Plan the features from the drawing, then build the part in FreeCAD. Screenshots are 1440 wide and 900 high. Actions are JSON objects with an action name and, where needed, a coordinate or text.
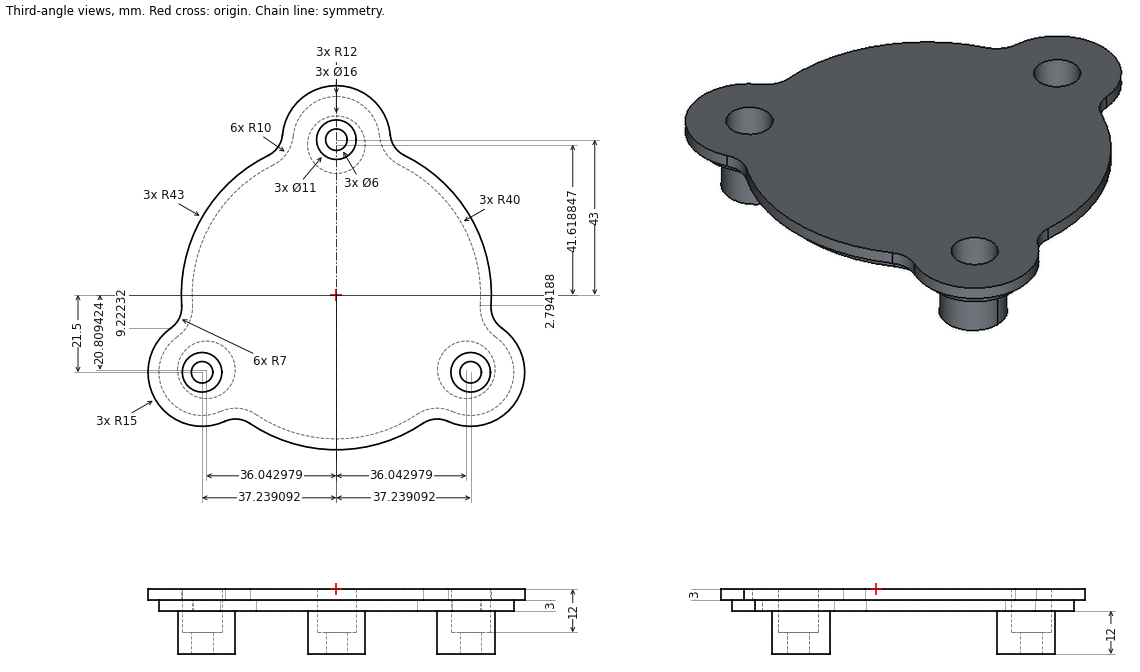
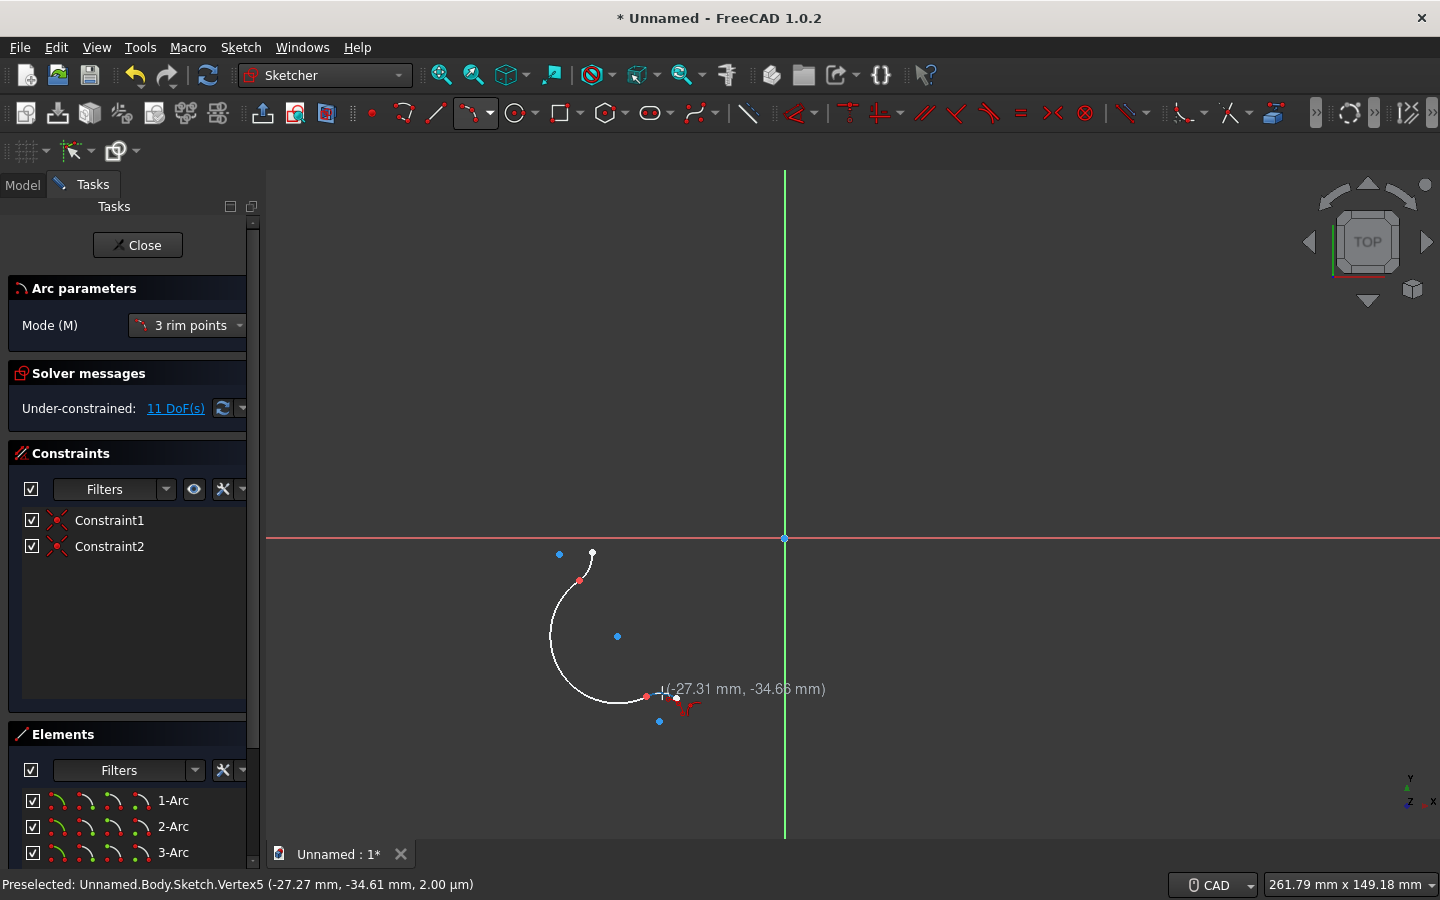
{"action": "left_click", "coordinate": [677, 699]}
{"action": "left_click", "coordinate": [893, 698]}
{"action": "left_click", "coordinate": [762, 730]}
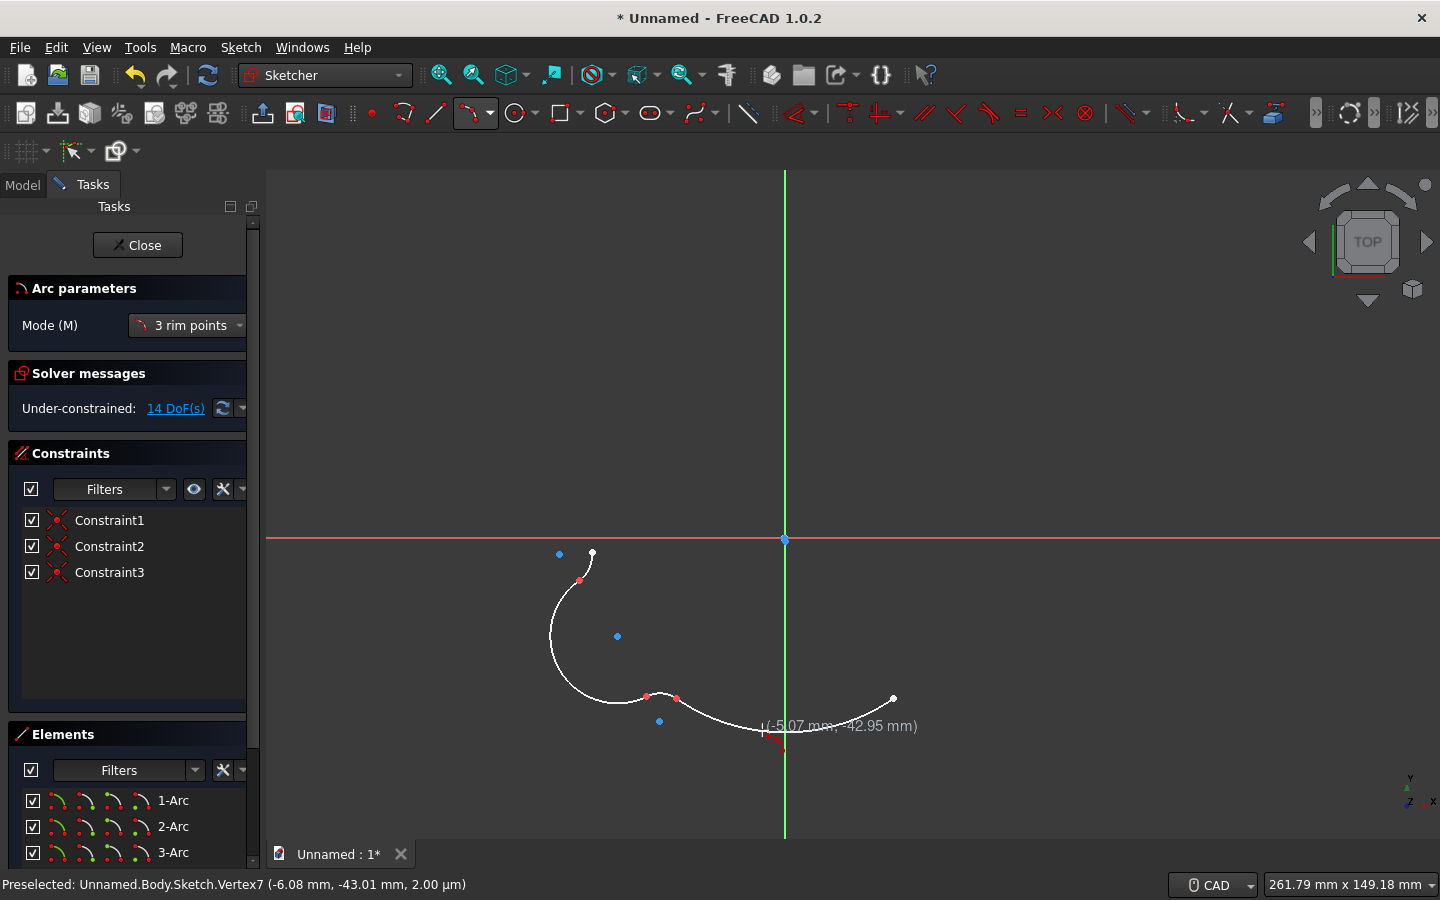
{"action": "left_click", "coordinate": [893, 699]}
{"action": "left_click", "coordinate": [923, 696]}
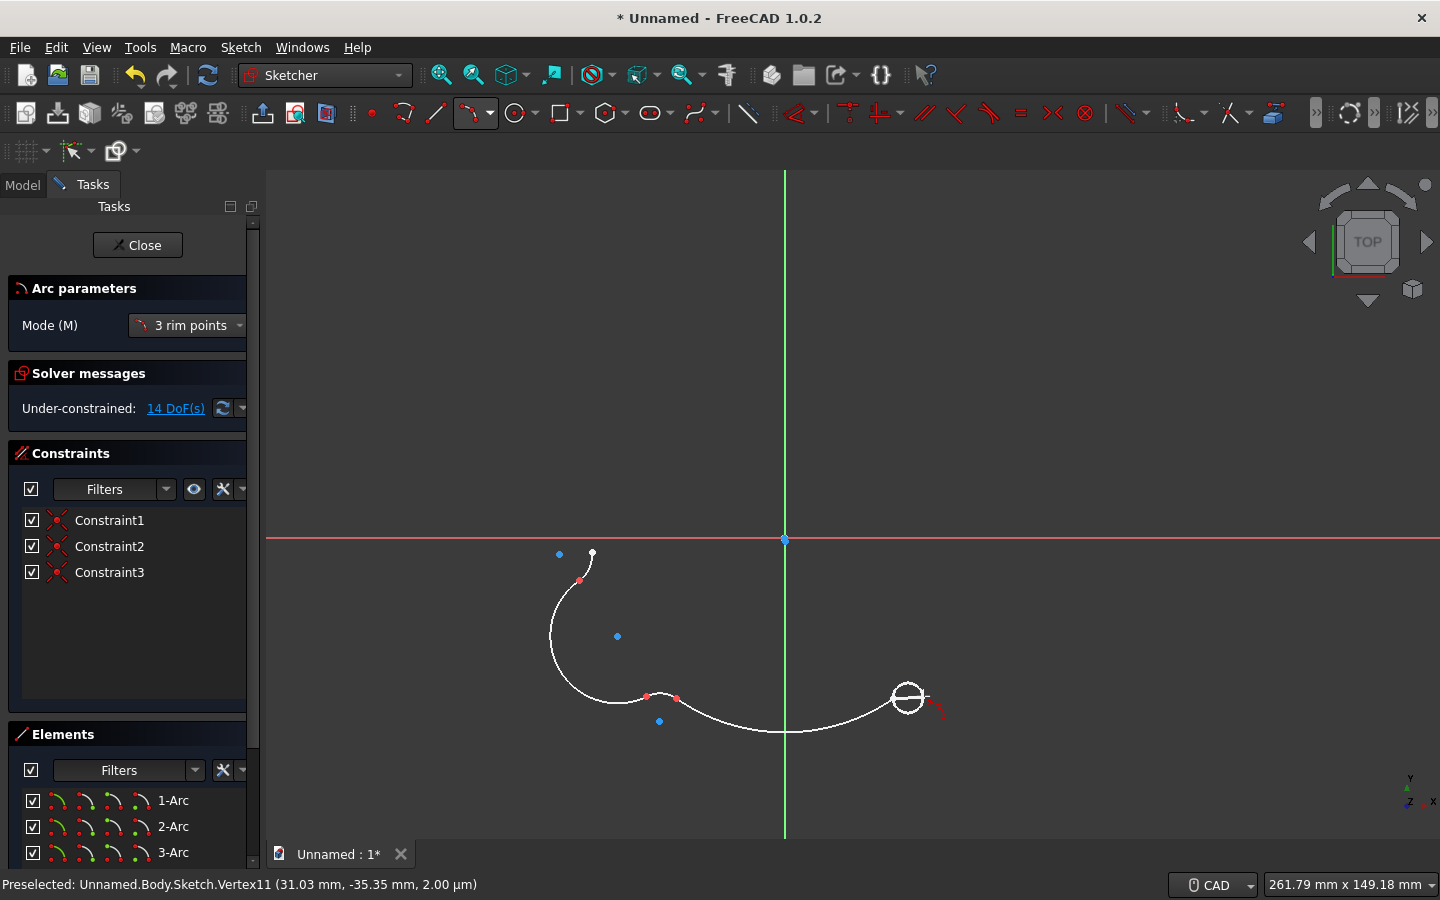
{"action": "scroll", "coordinate": [908, 693], "scroll_direction": "up", "scroll_amount": 7}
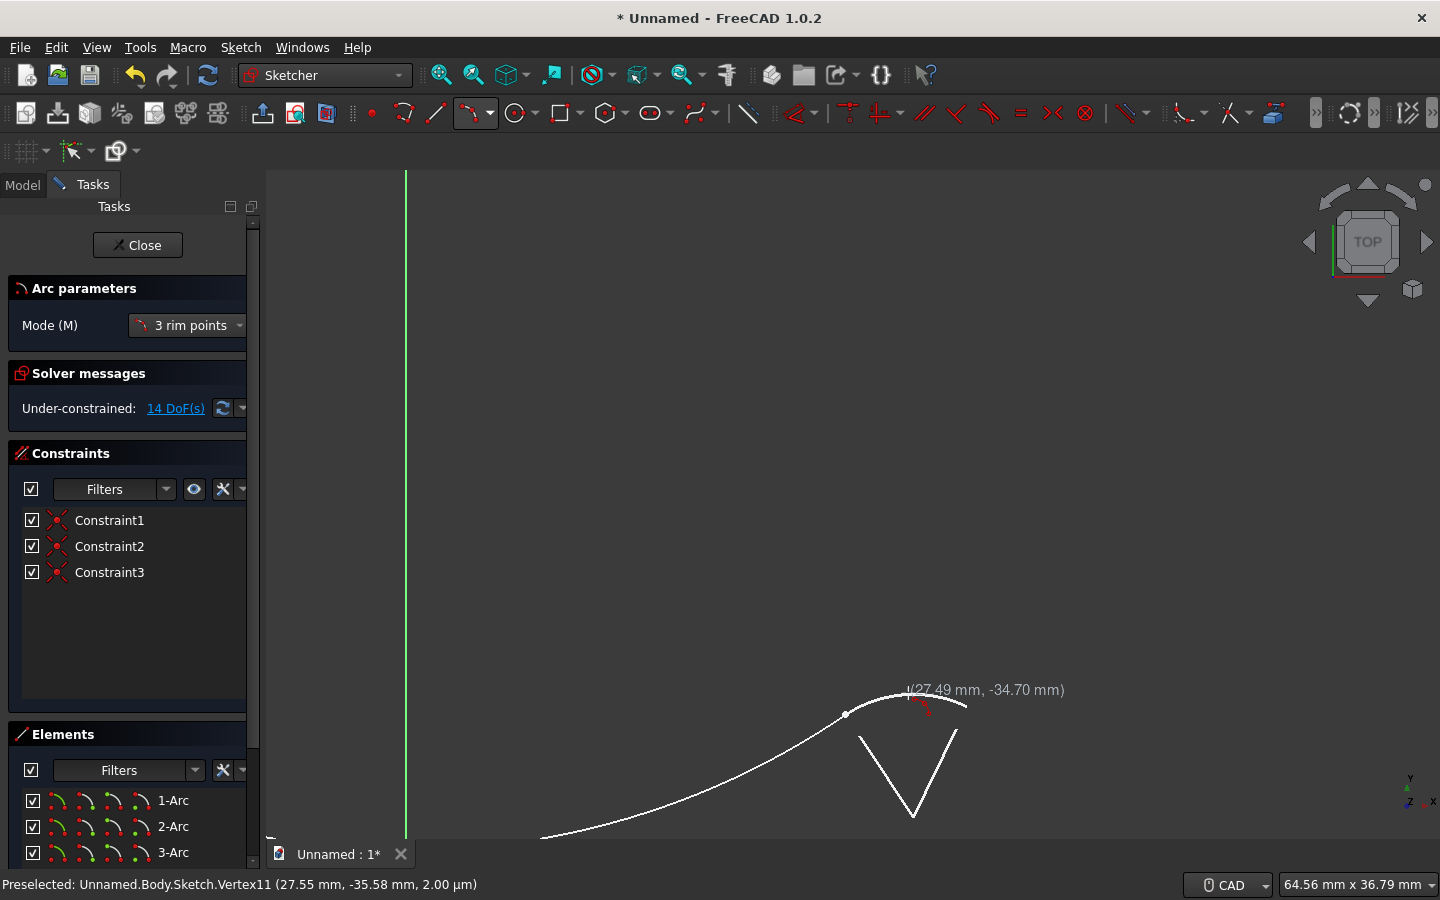
{"action": "left_click", "coordinate": [905, 691]}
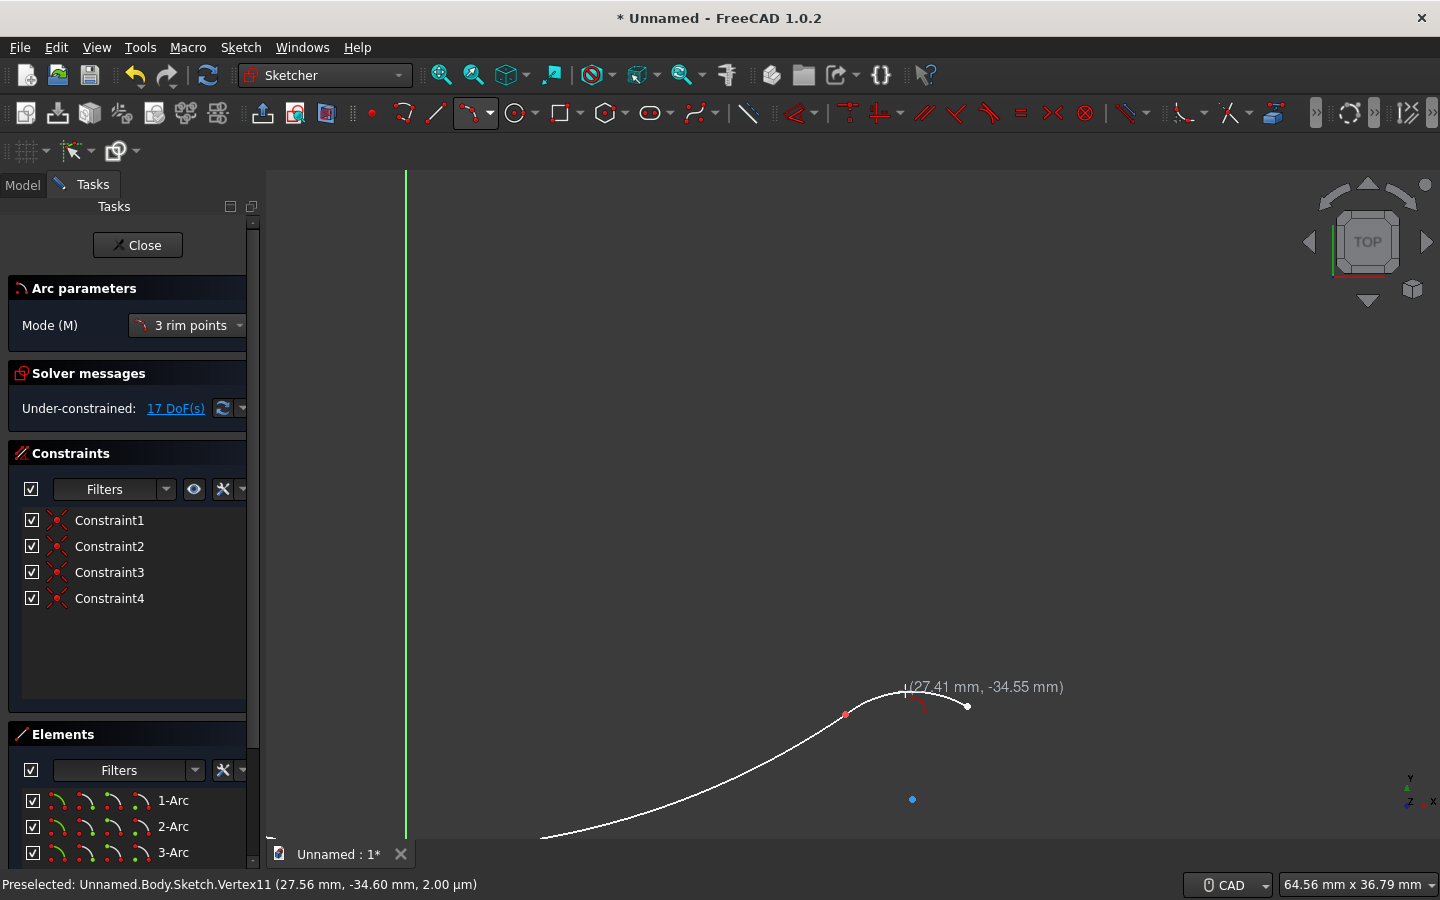
{"action": "scroll", "coordinate": [908, 693], "scroll_direction": "down", "scroll_amount": 7}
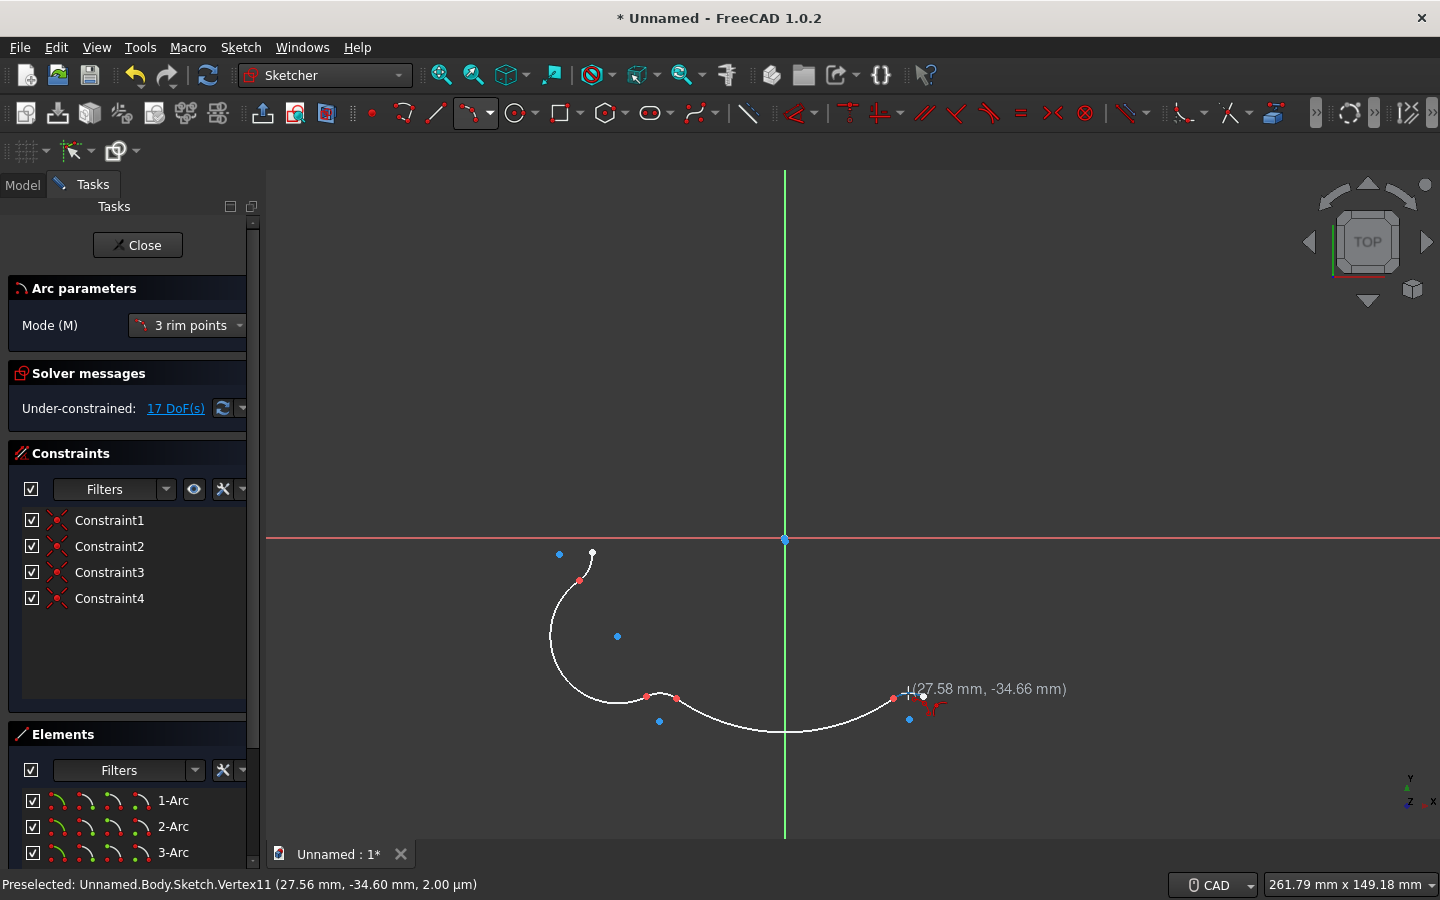
{"action": "left_click", "coordinate": [923, 697]}
{"action": "left_click", "coordinate": [990, 580]}
{"action": "left_click", "coordinate": [1010, 668]}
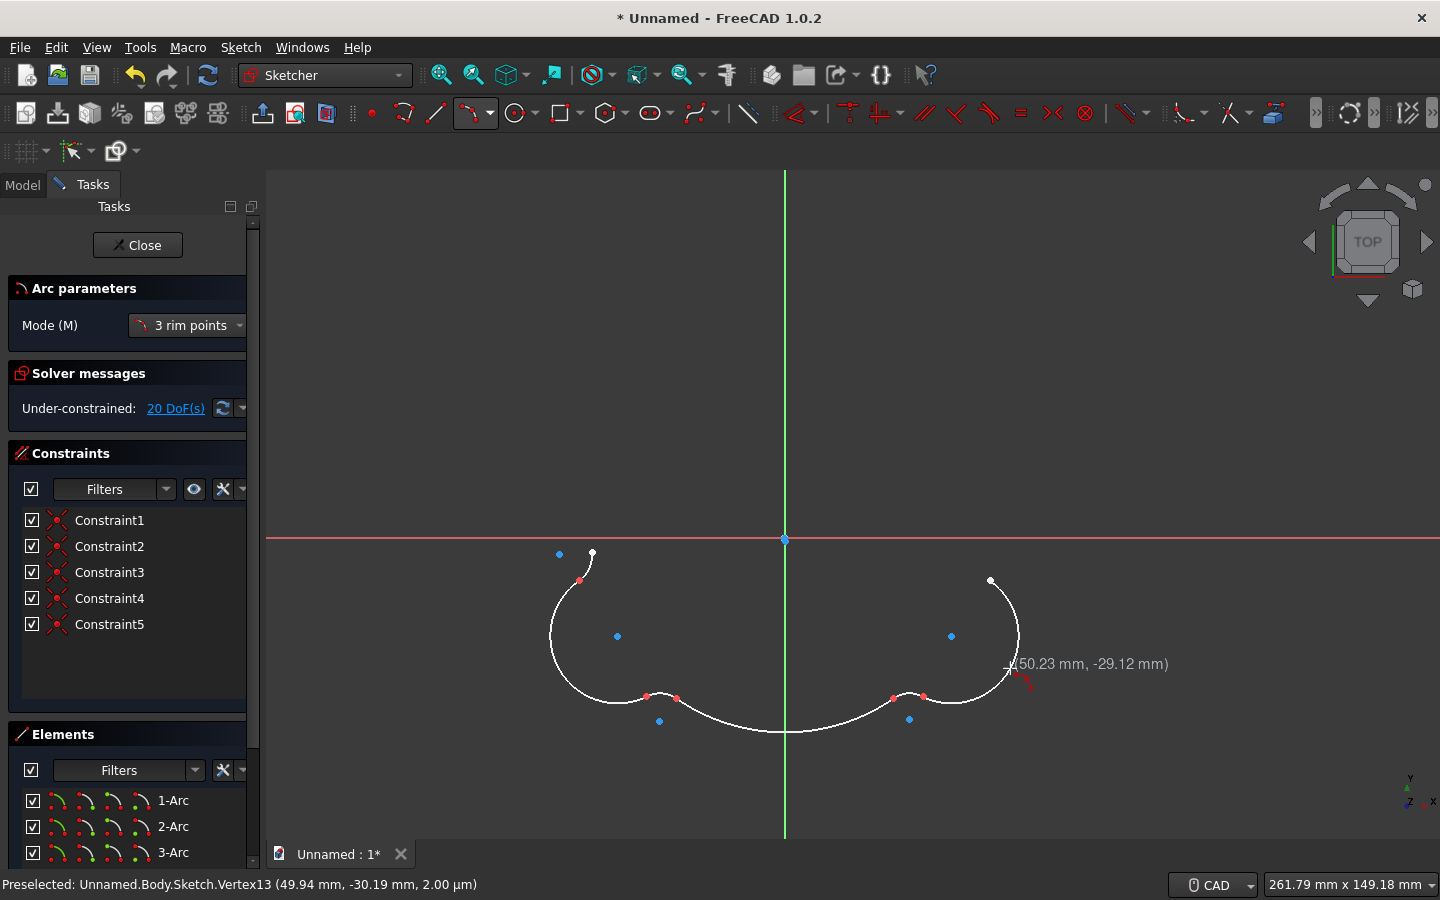
{"action": "left_click", "coordinate": [990, 581]}
{"action": "left_click", "coordinate": [977, 552]}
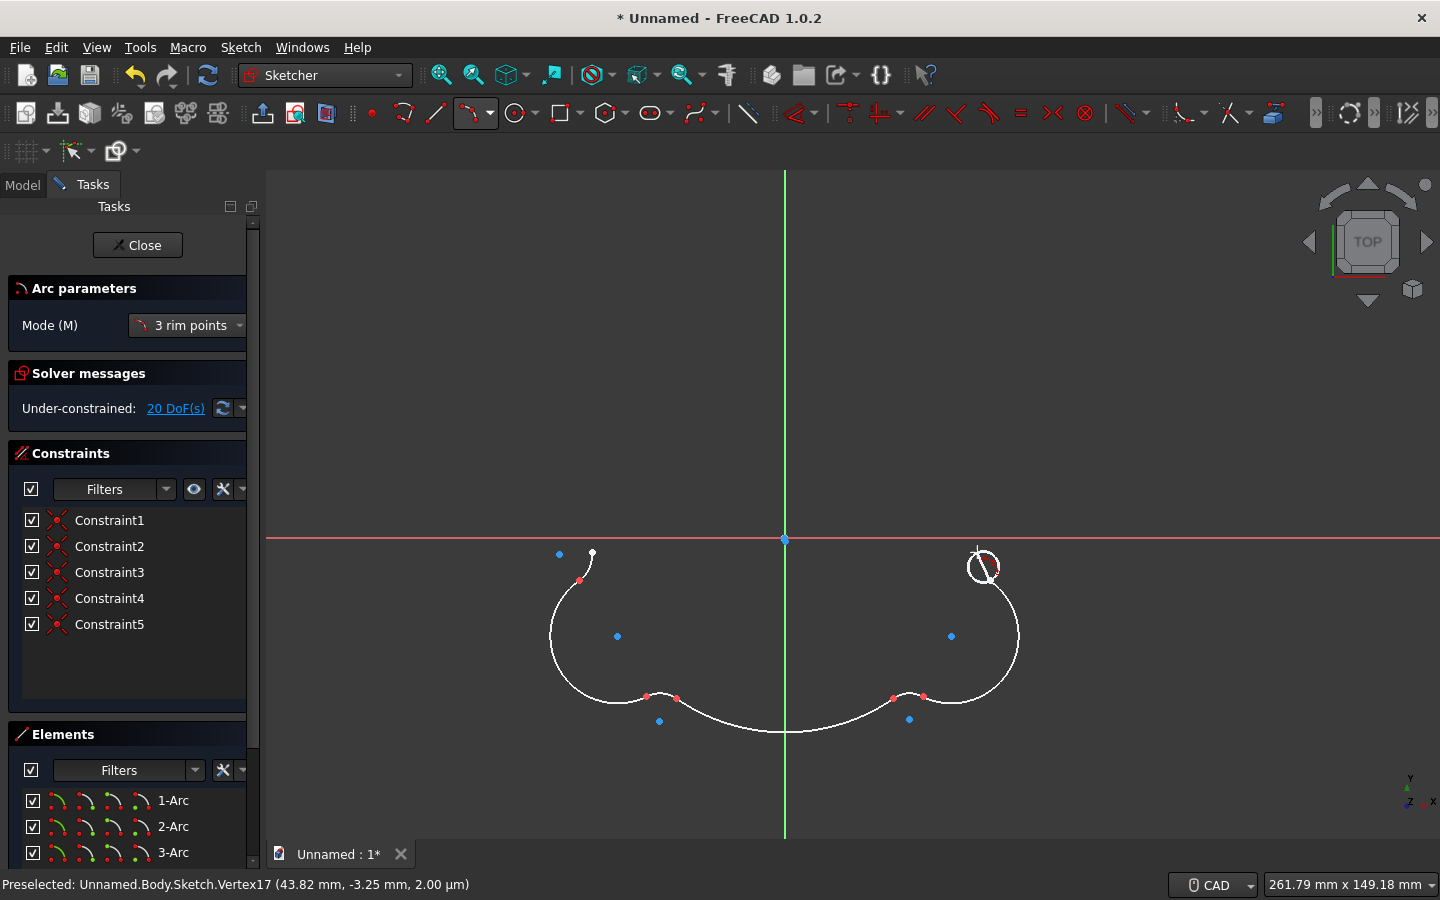
{"action": "scroll", "coordinate": [980, 568], "scroll_direction": "up", "scroll_amount": 7}